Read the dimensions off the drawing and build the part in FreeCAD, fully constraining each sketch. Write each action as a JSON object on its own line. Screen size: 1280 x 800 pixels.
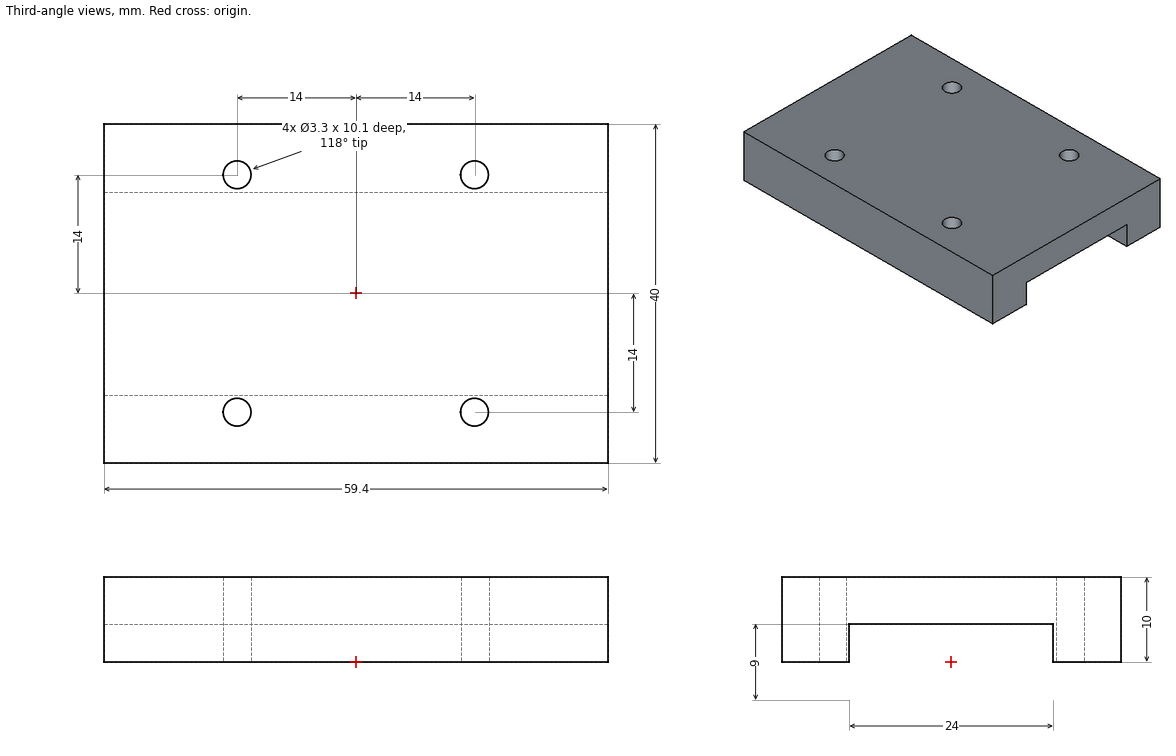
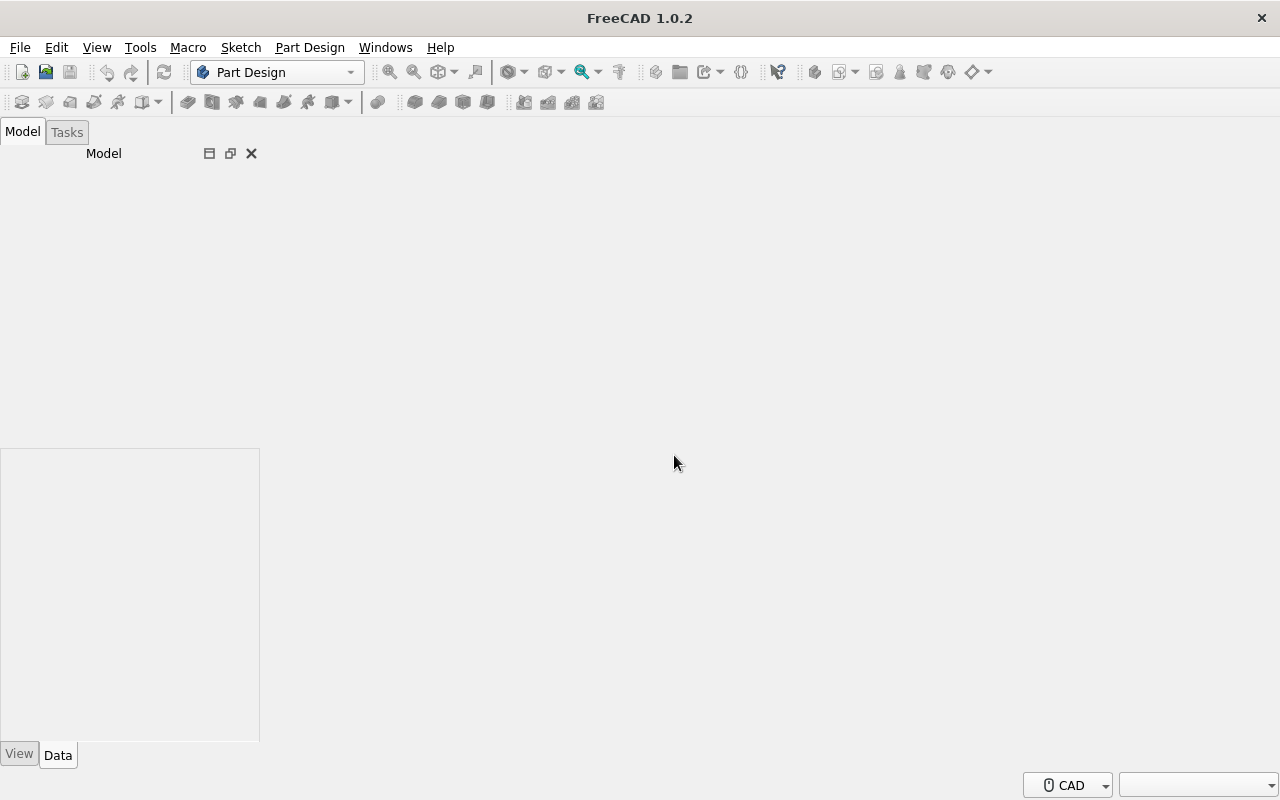
{"action": "key", "text": "ctrl+n"}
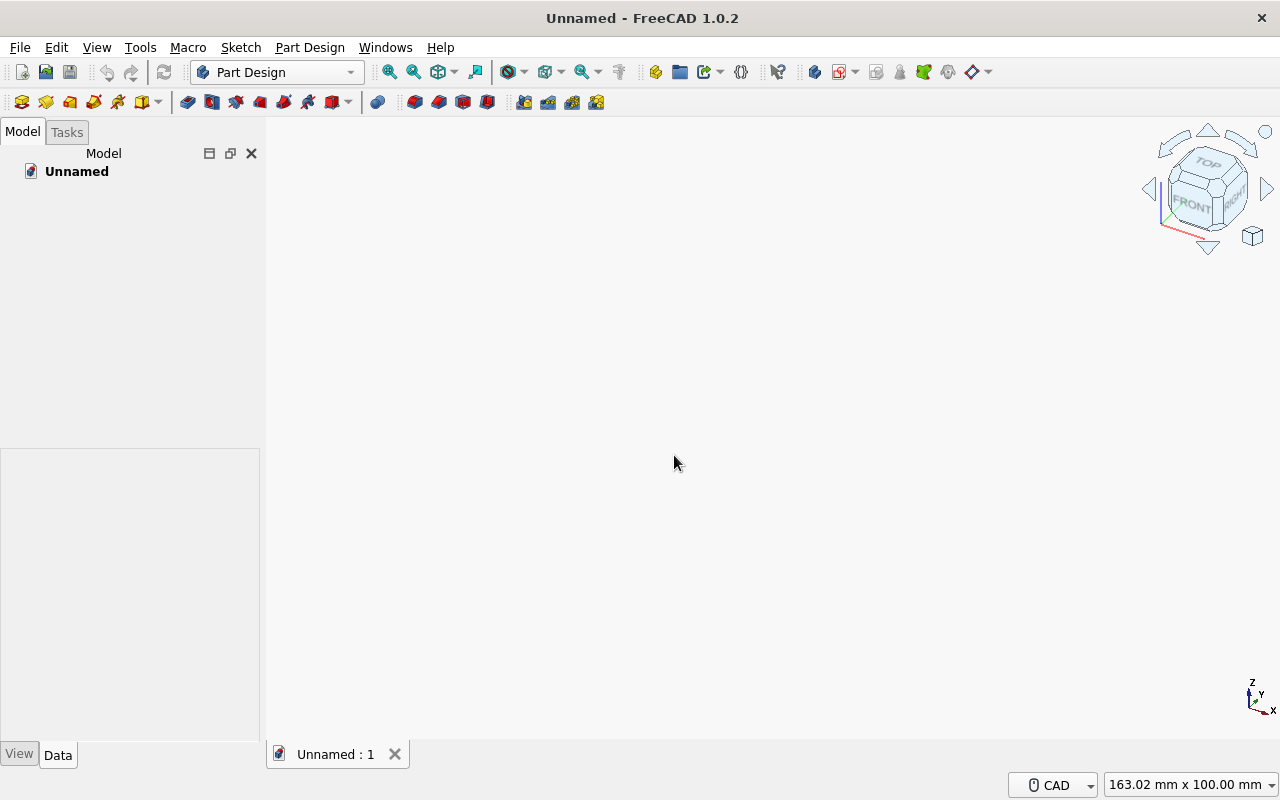
{"action": "left_click", "coordinate": [840, 72]}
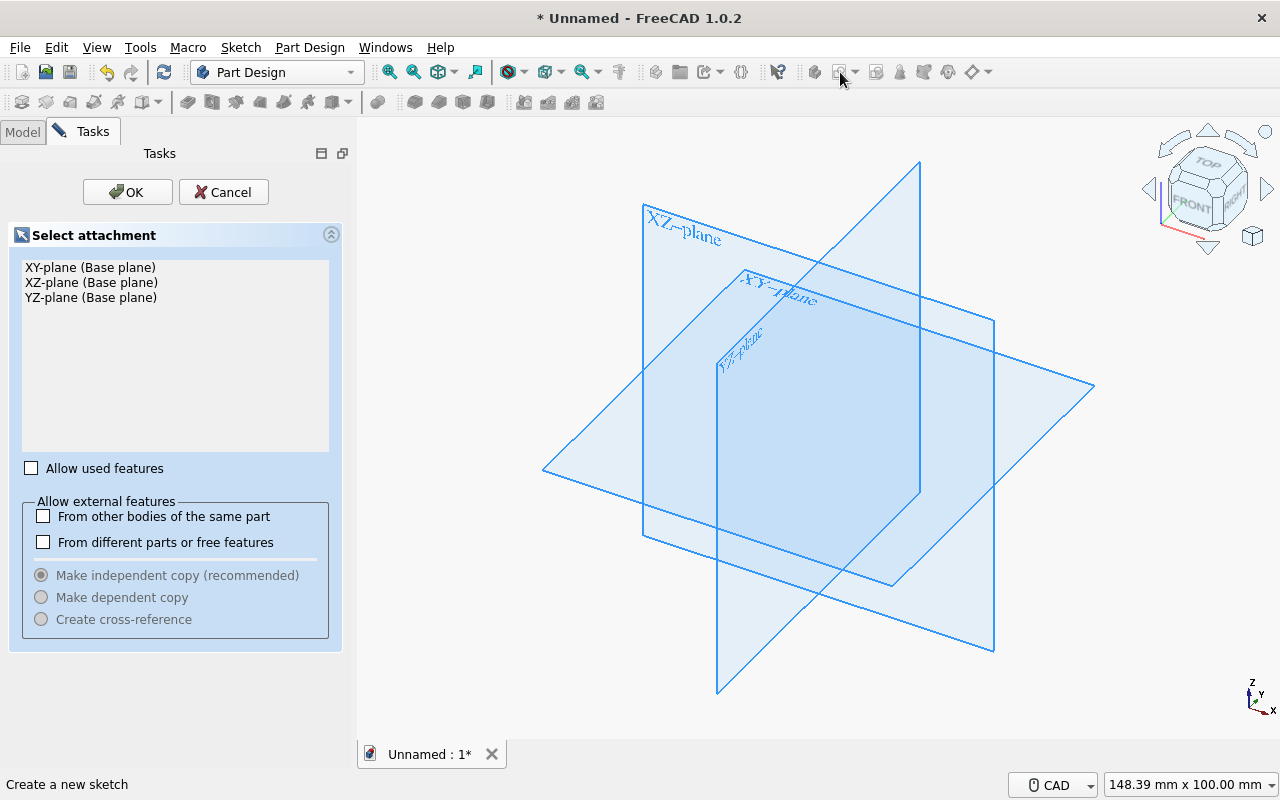
{"action": "left_click", "coordinate": [82, 268]}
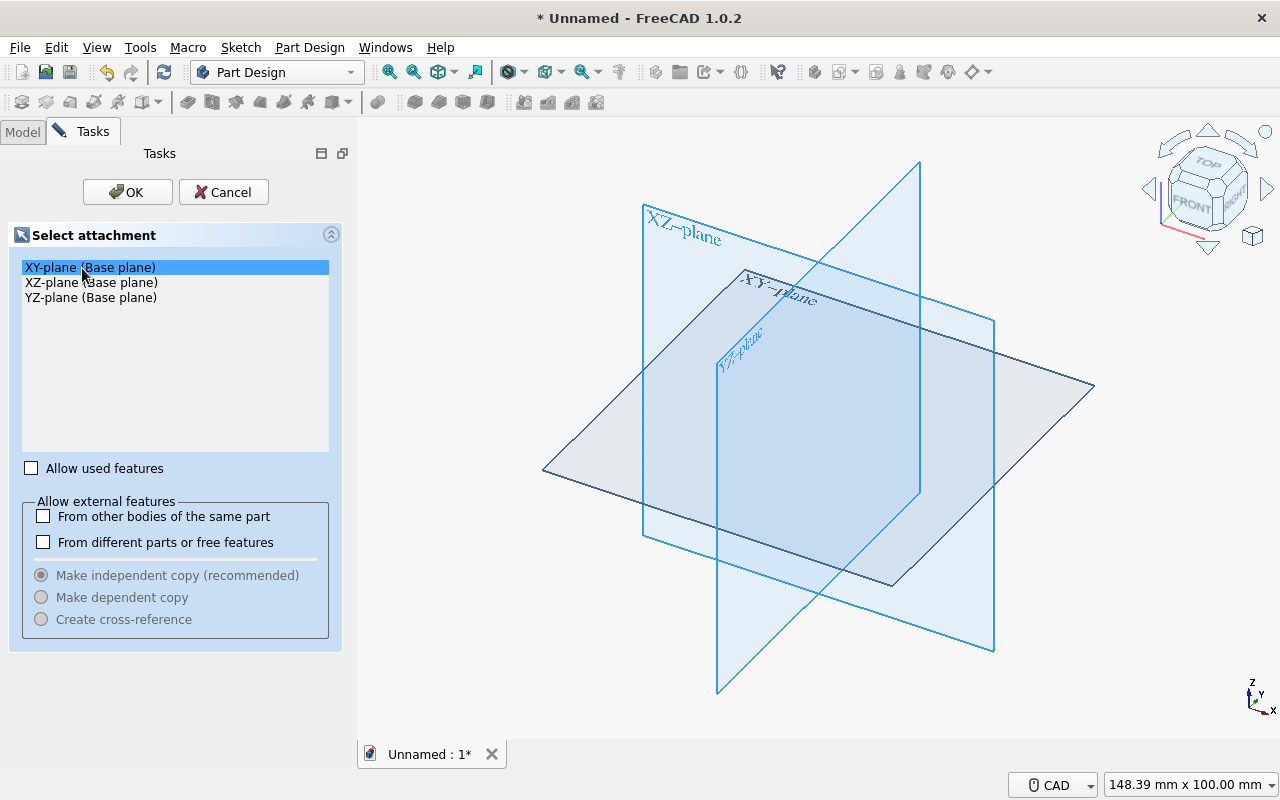
{"action": "left_click", "coordinate": [128, 192]}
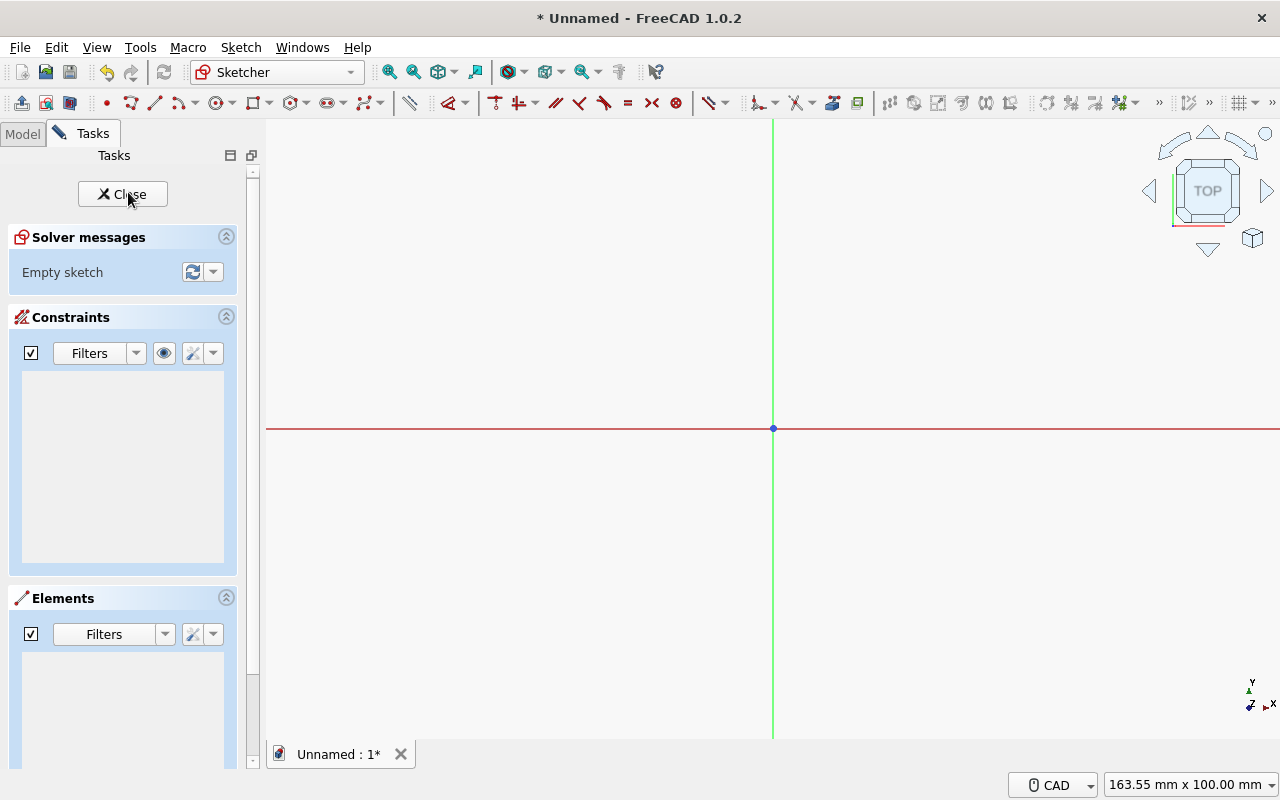
{"action": "scroll", "coordinate": [912, 429], "scroll_direction": "up", "scroll_amount": 2}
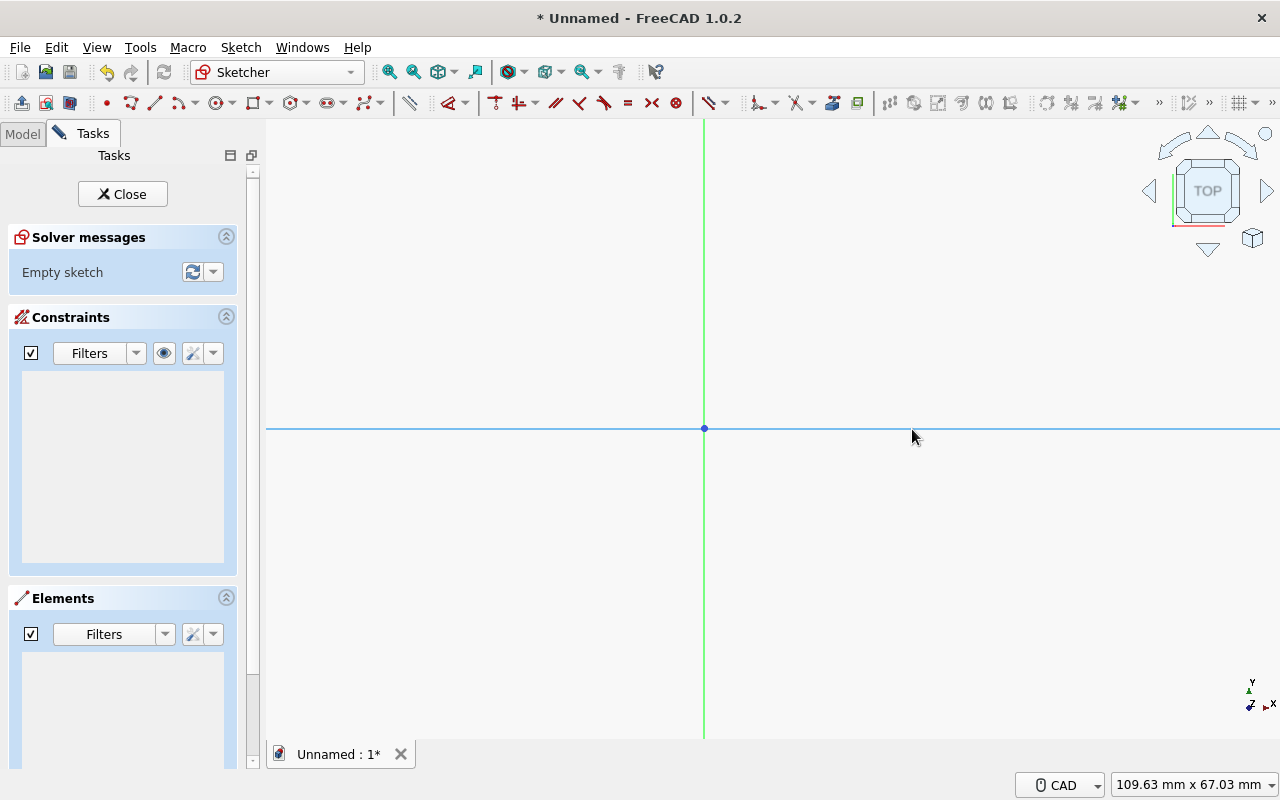
{"action": "key", "text": "g v"}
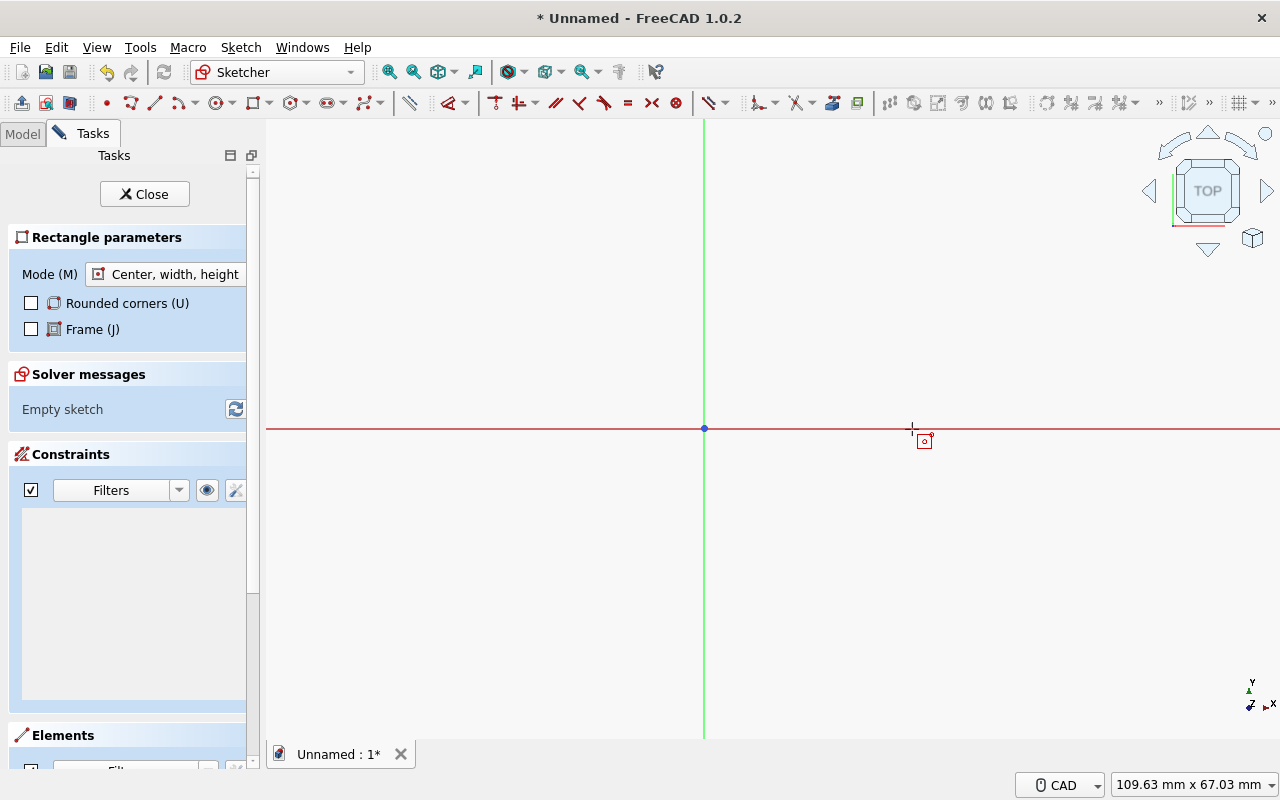
{"action": "left_click", "coordinate": [704, 429]}
{"action": "left_click", "coordinate": [979, 244]}
{"action": "key", "text": "Escape"}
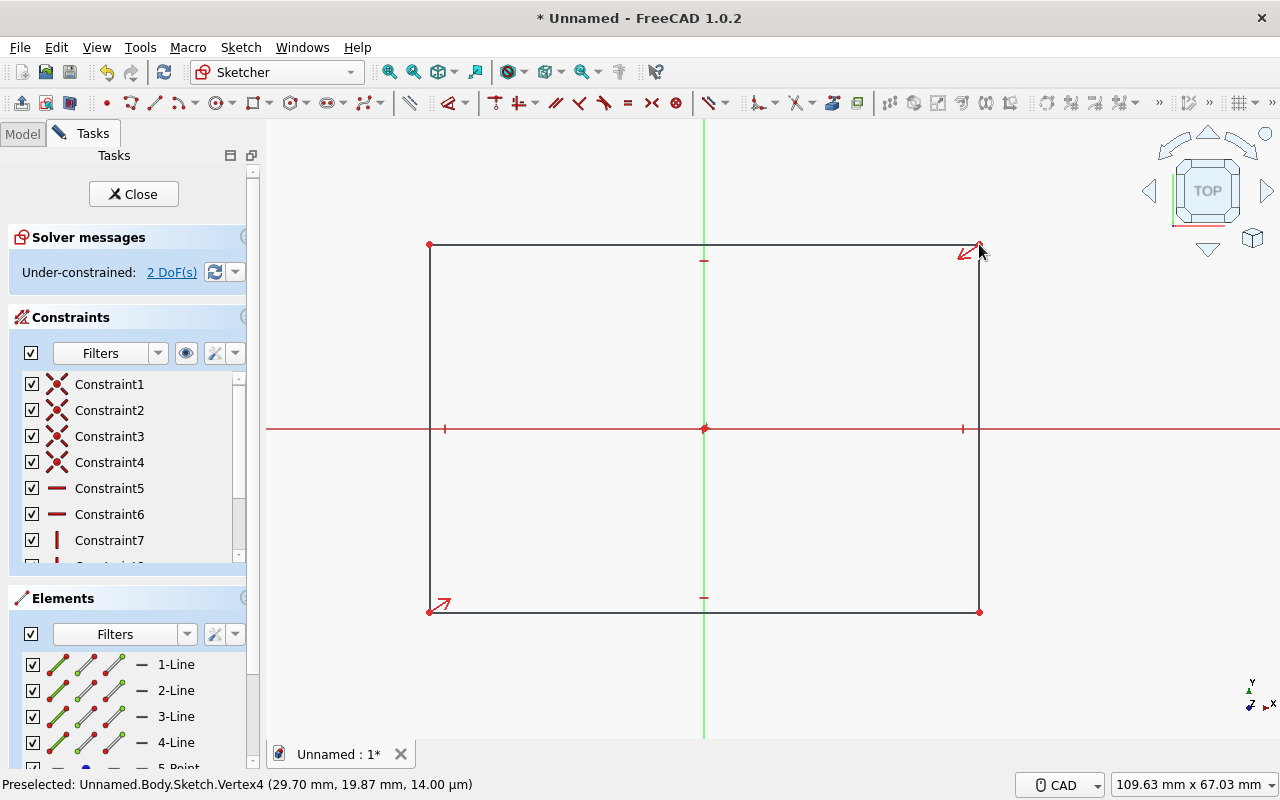
{"action": "left_click", "coordinate": [448, 104]}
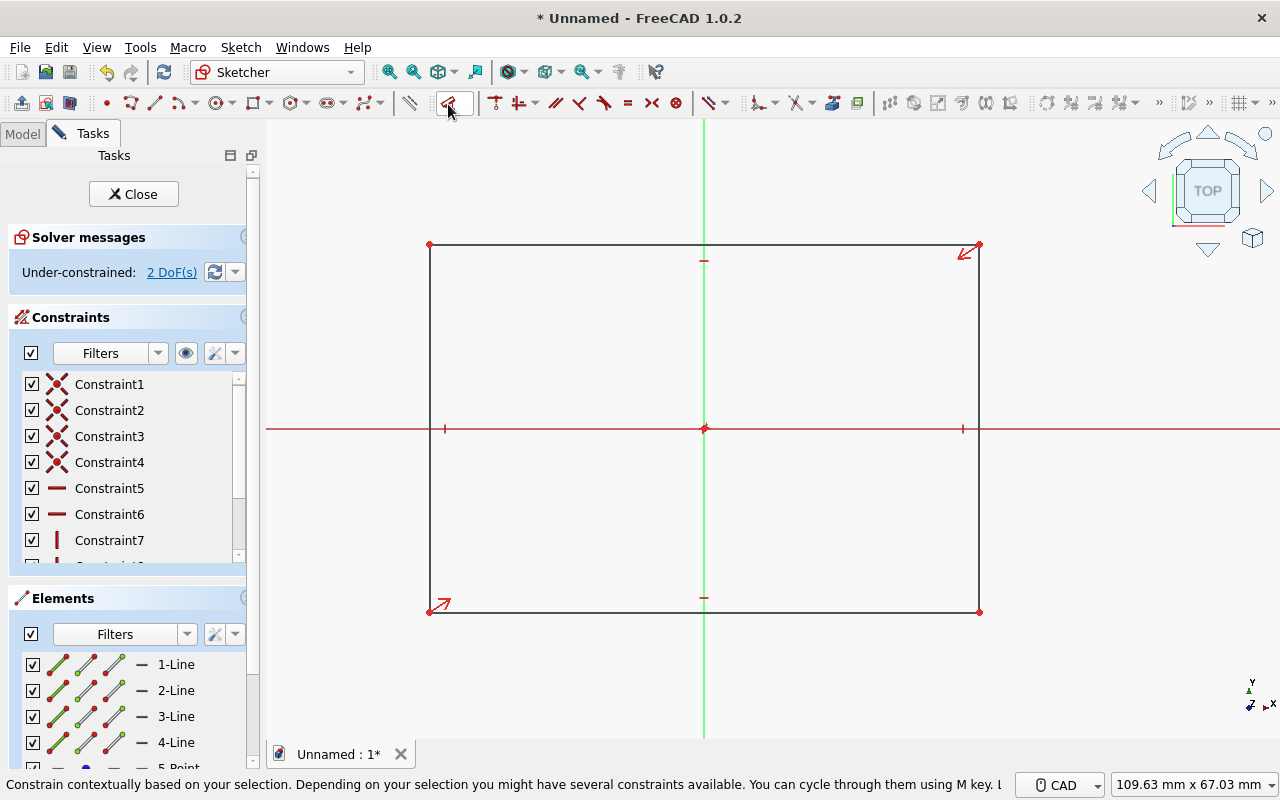
{"action": "left_click", "coordinate": [979, 502]}
{"action": "left_click", "coordinate": [1013, 344]}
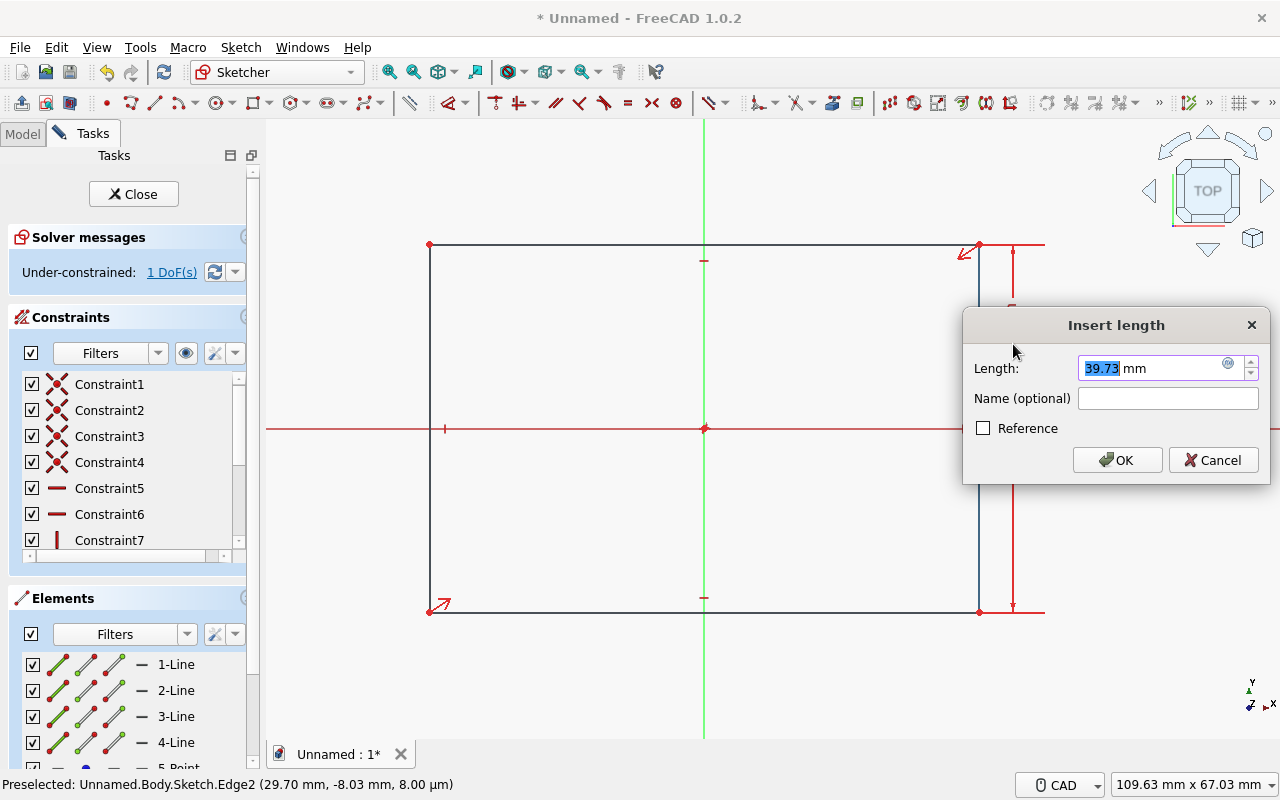
{"action": "type", "text": "40"}
{"action": "key", "text": "Return"}